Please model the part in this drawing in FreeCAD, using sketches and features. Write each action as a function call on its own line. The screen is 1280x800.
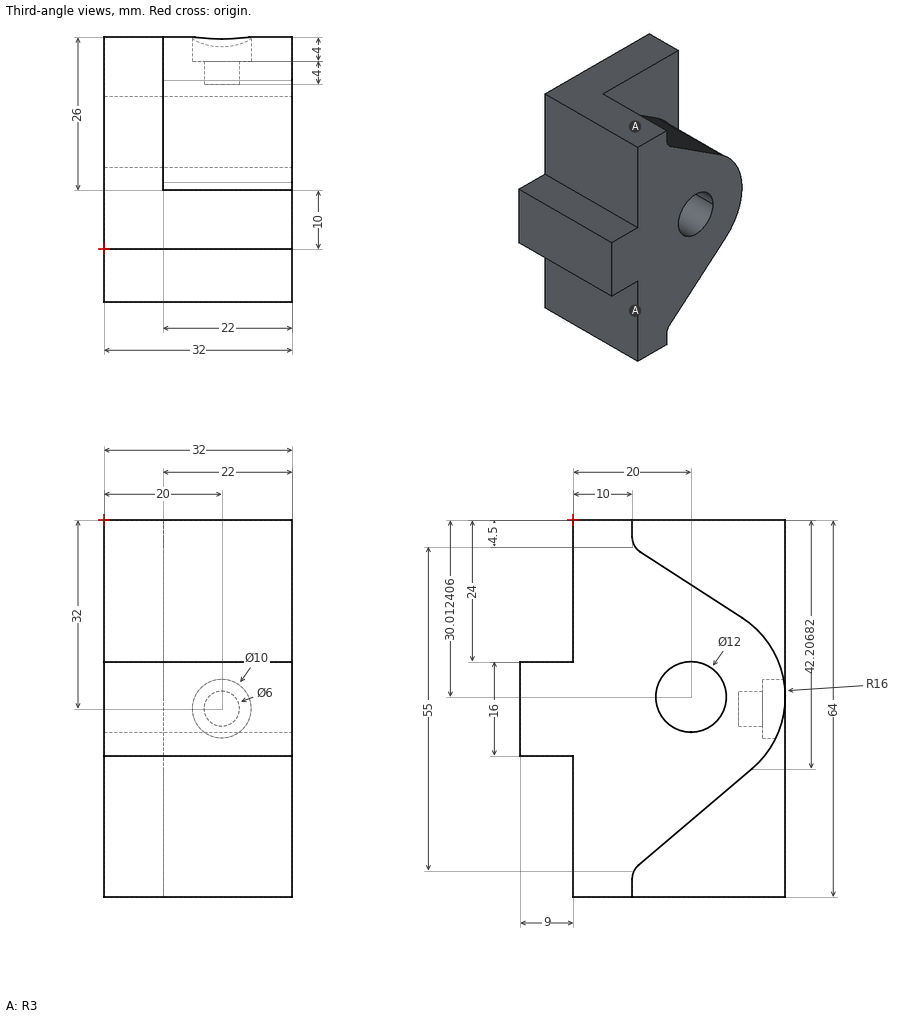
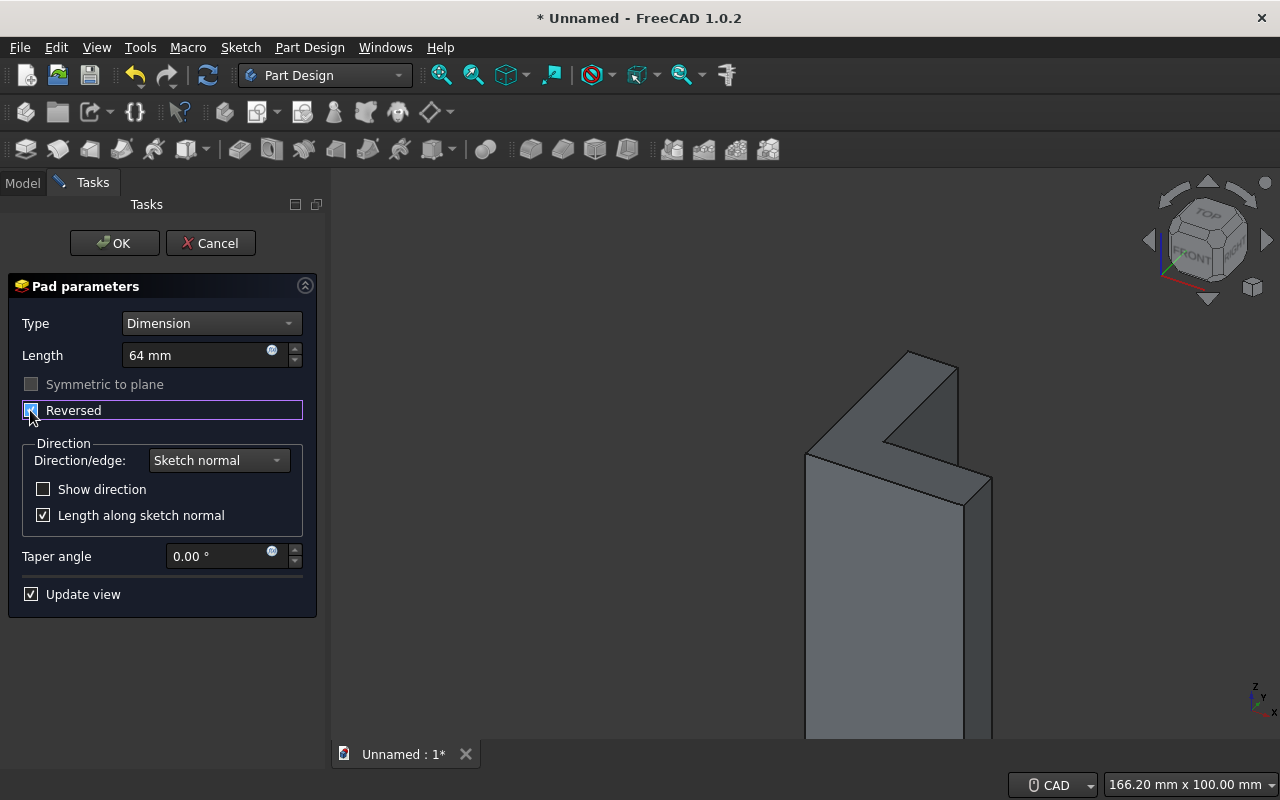
click(115, 243)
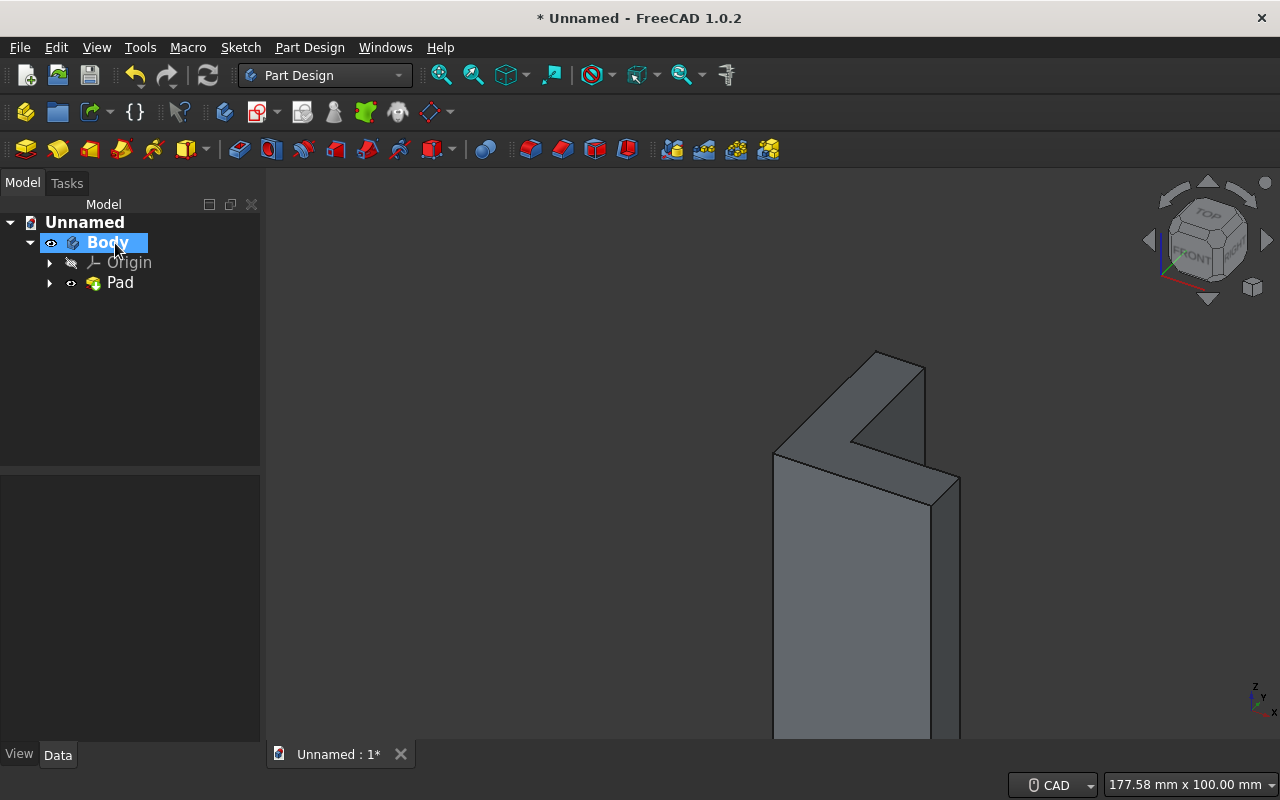
click(442, 76)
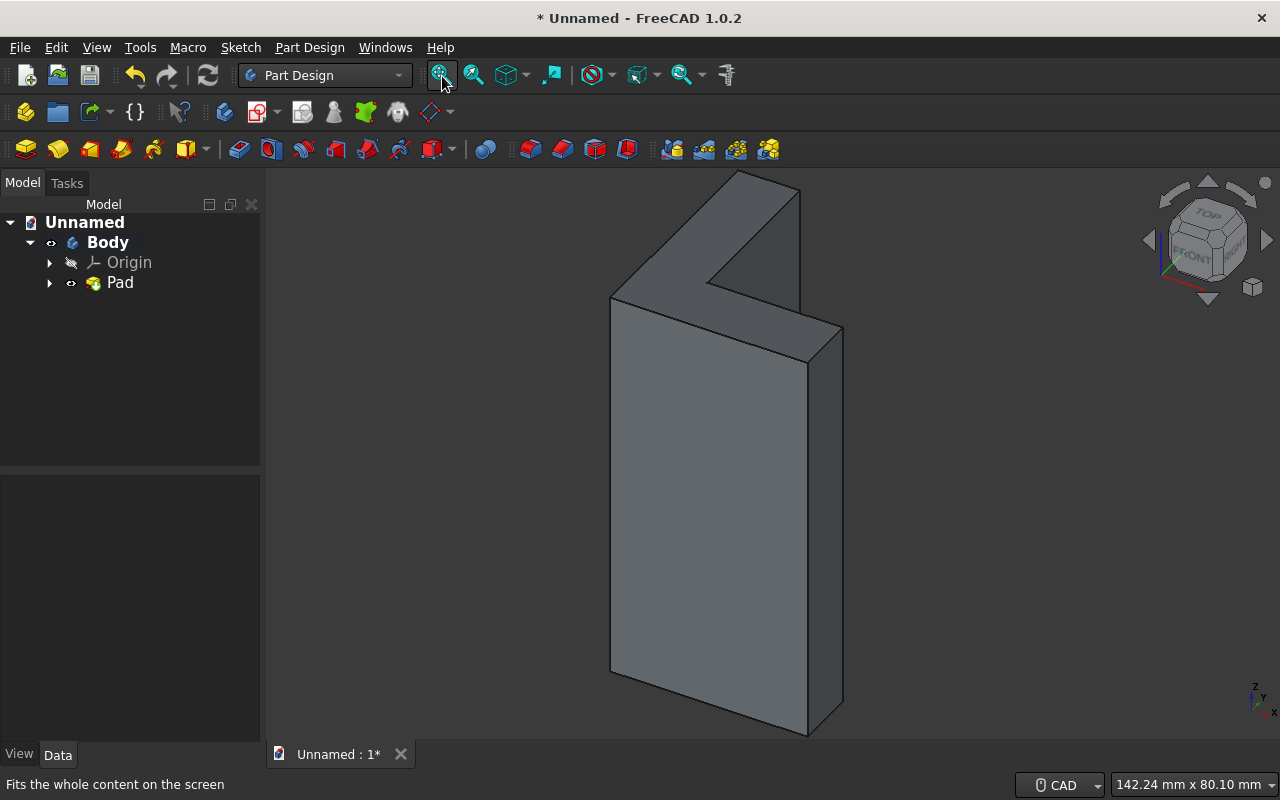
click(825, 424)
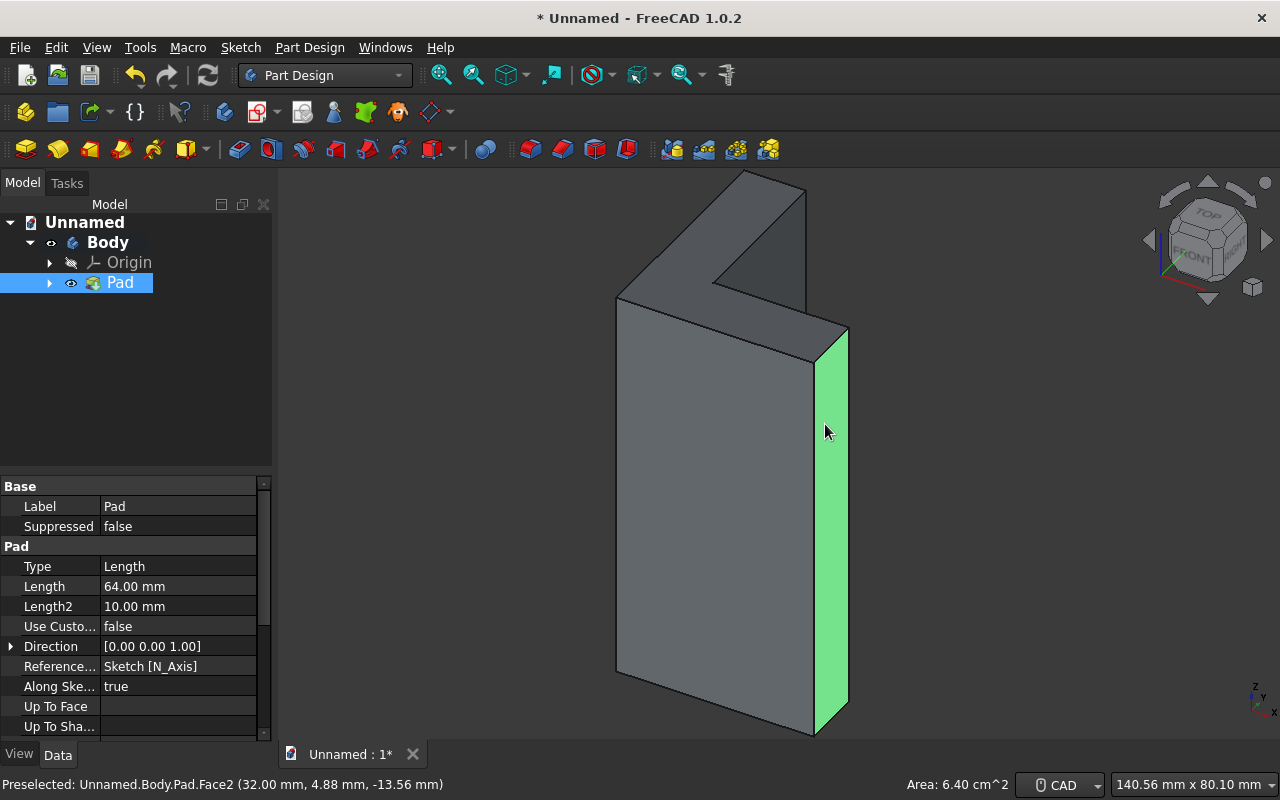
click(258, 112)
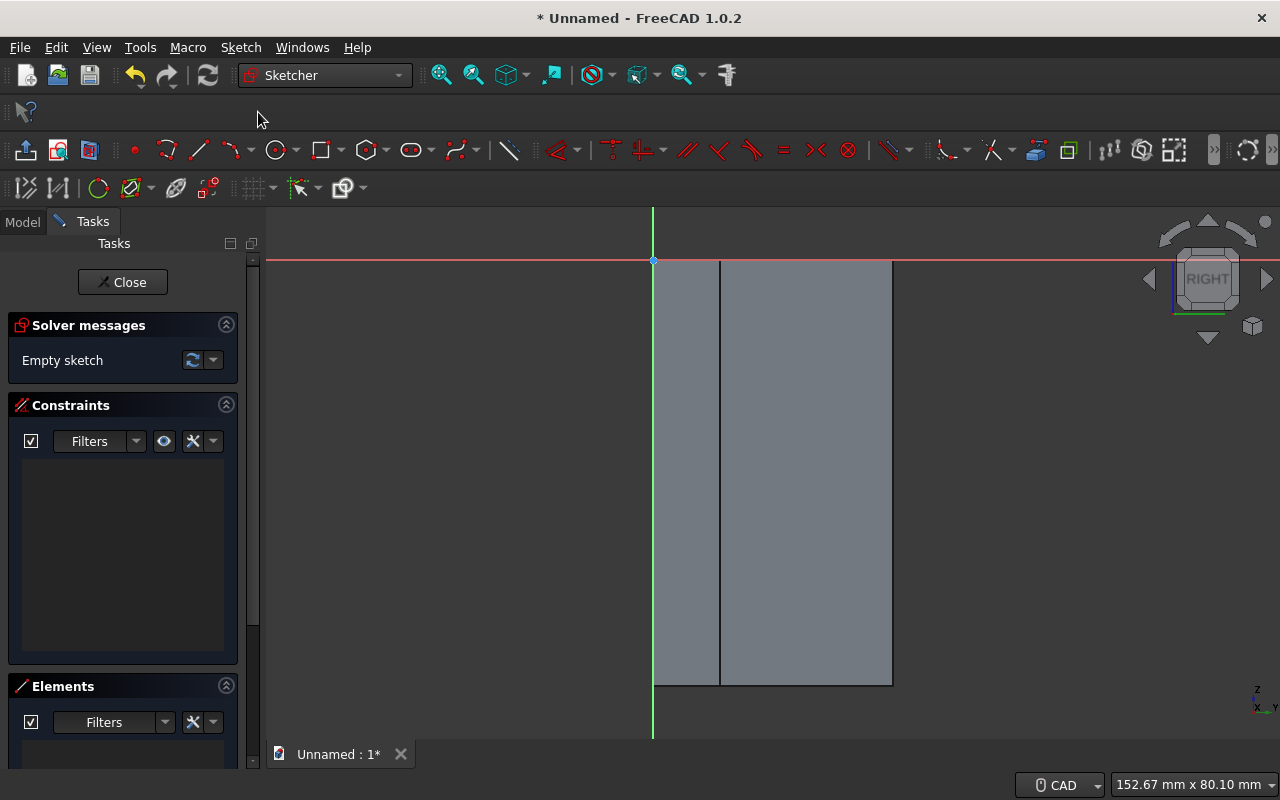
key(g)
key(m)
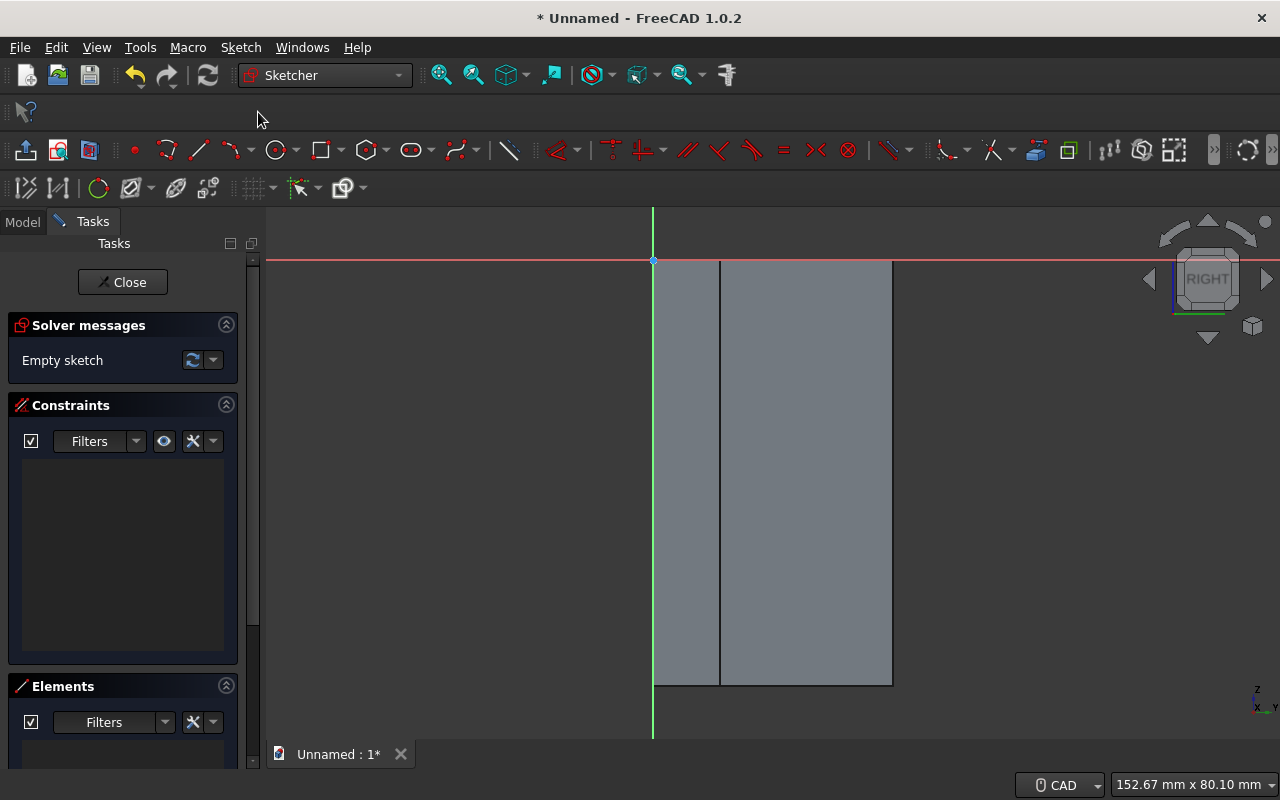
click(844, 371)
click(720, 290)
click(720, 656)
click(855, 541)
right_click(855, 541)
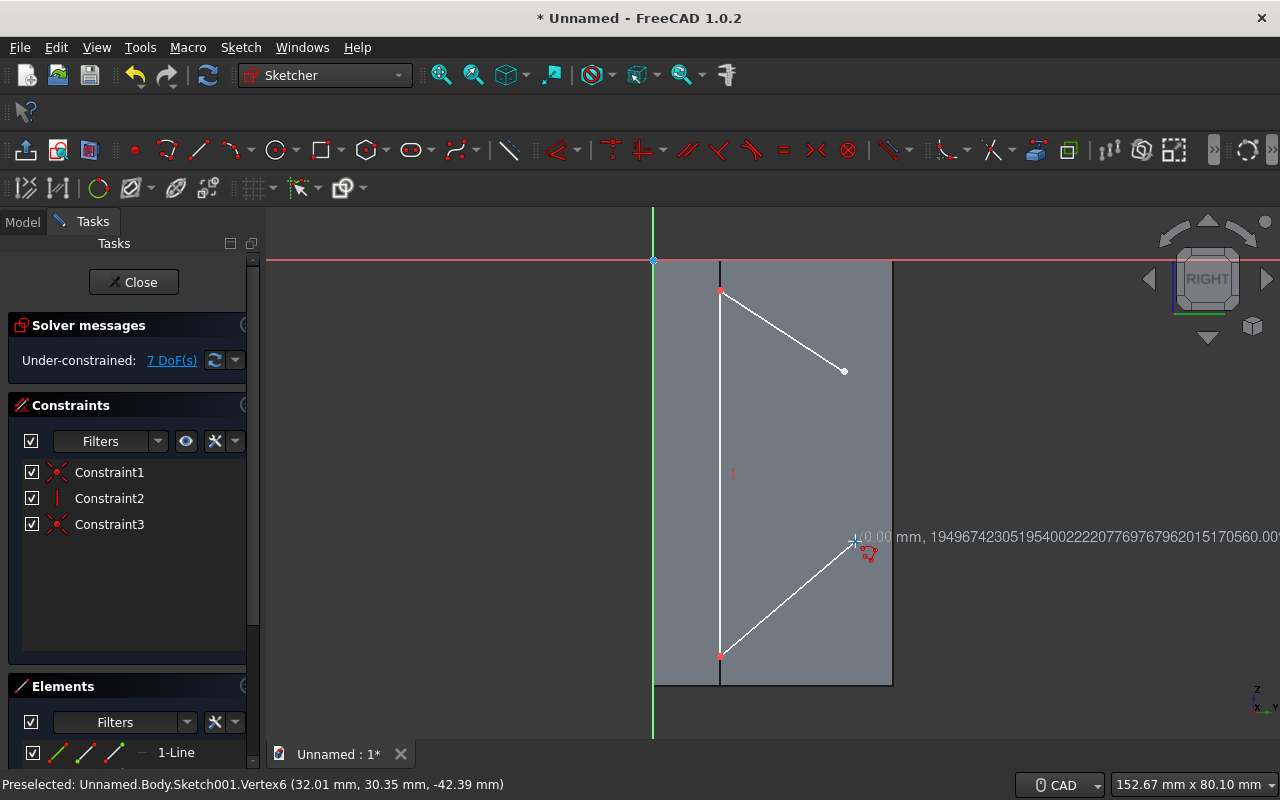
key(g)
key(3)
key(a)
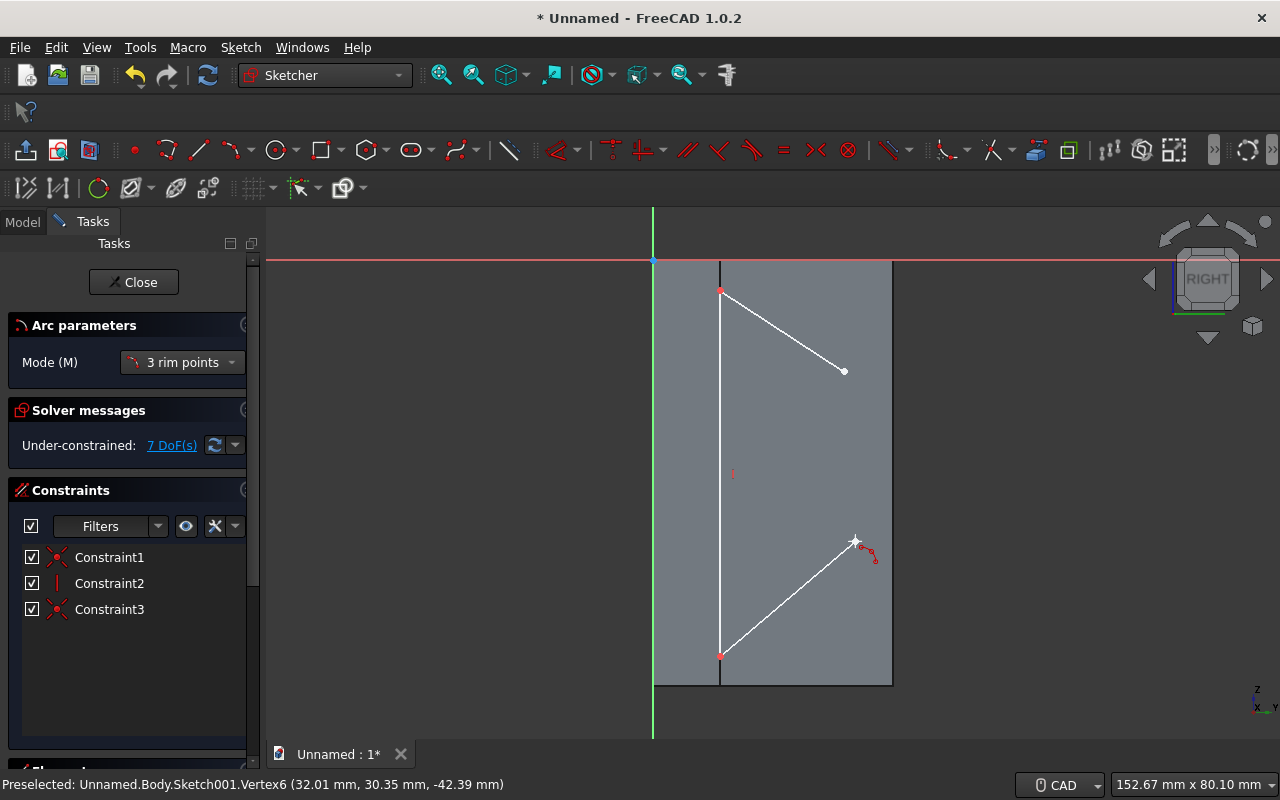
click(855, 542)
click(844, 372)
click(892, 453)
key(Escape)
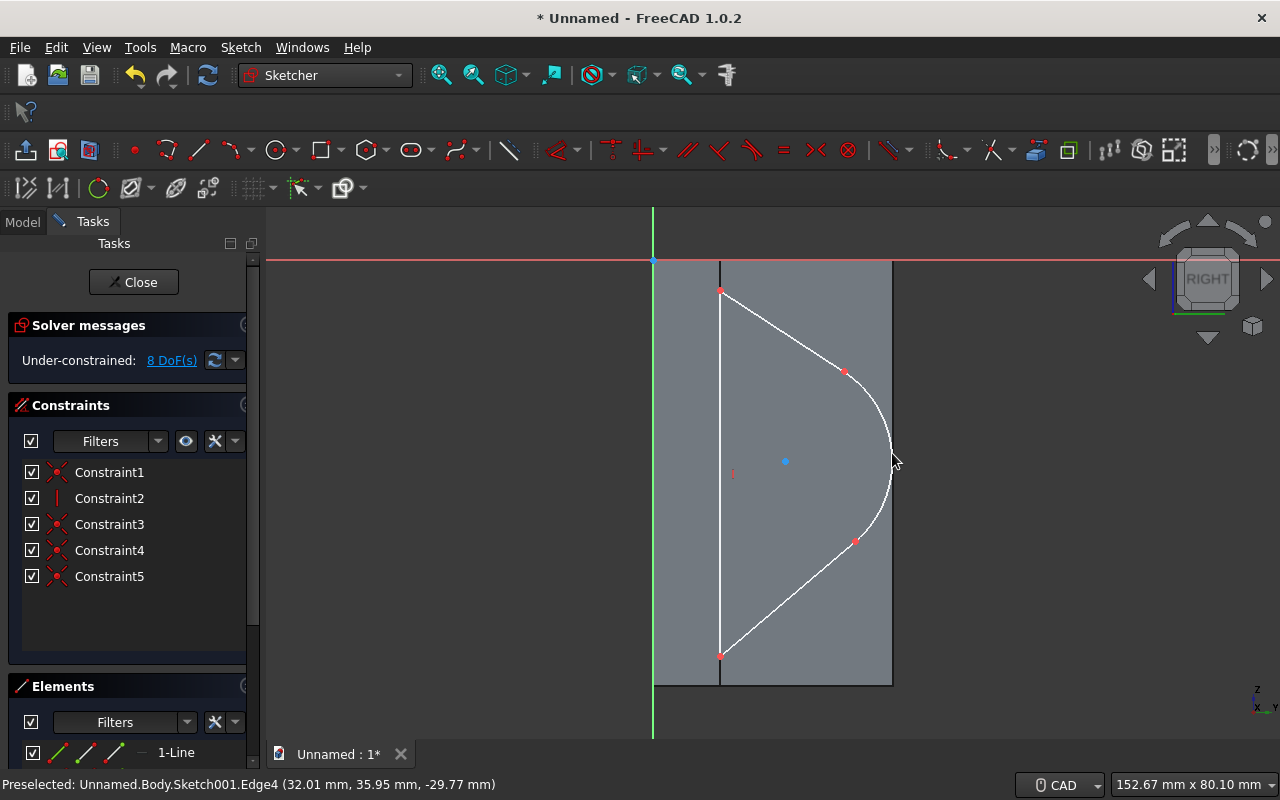
click(807, 348)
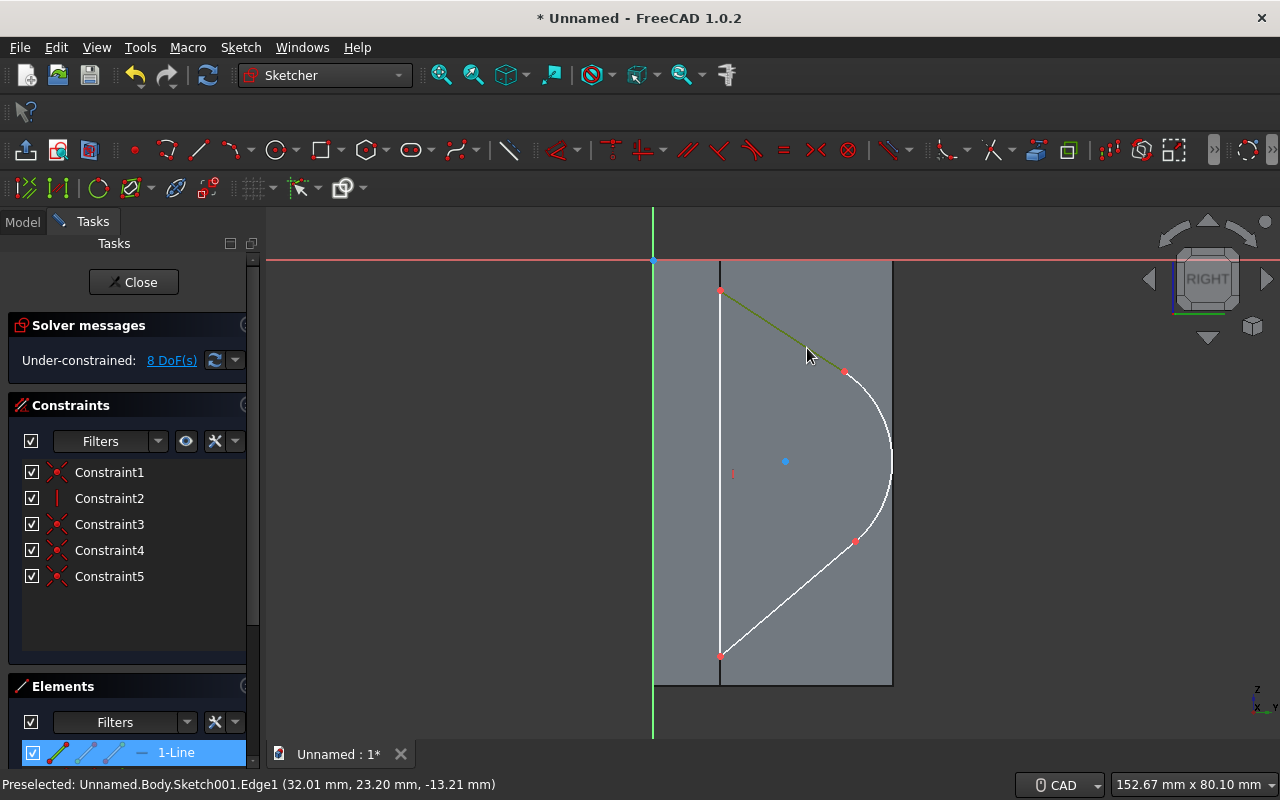
click(887, 493)